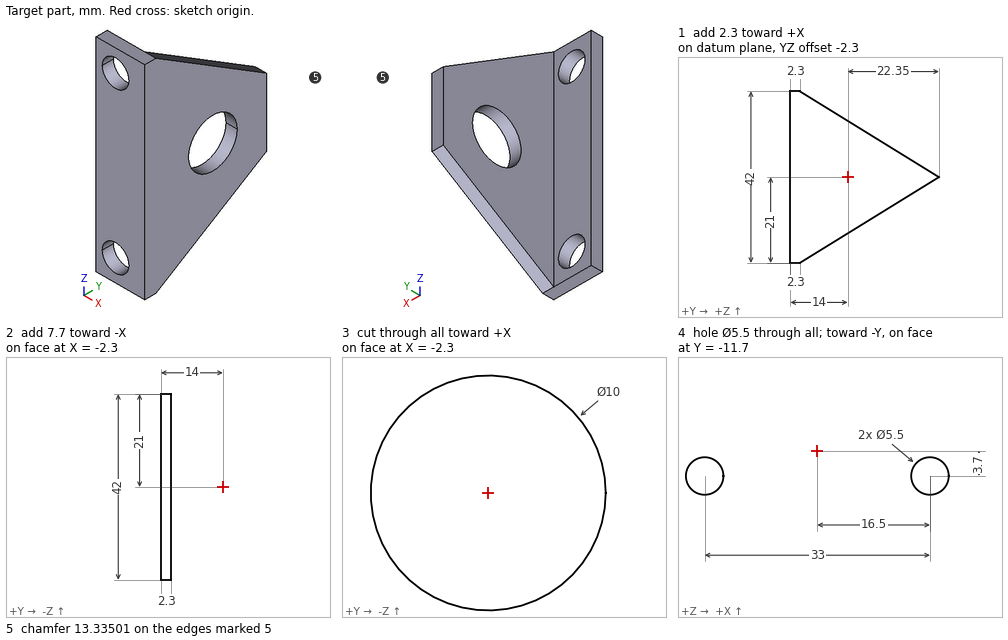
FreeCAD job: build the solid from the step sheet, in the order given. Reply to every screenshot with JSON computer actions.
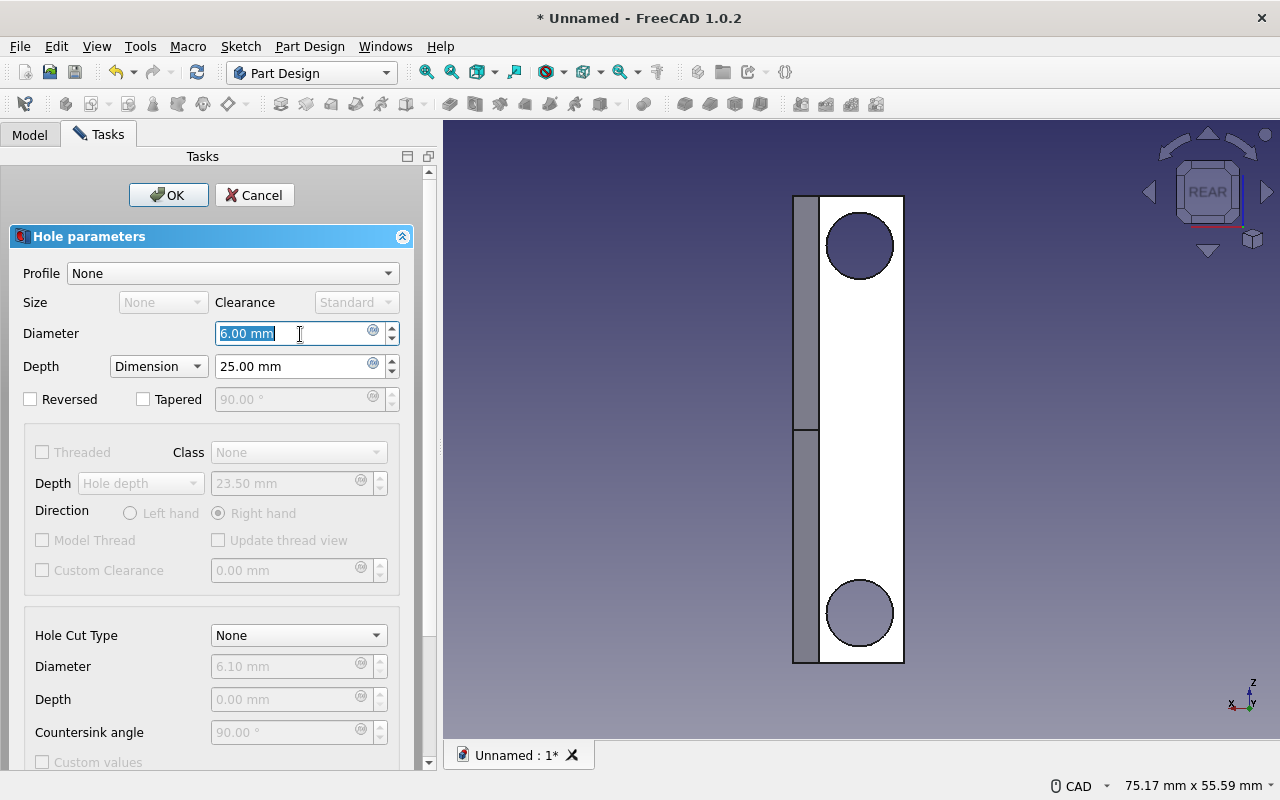
{"action": "type", "text": "5.5"}
{"action": "key", "text": "Tab"}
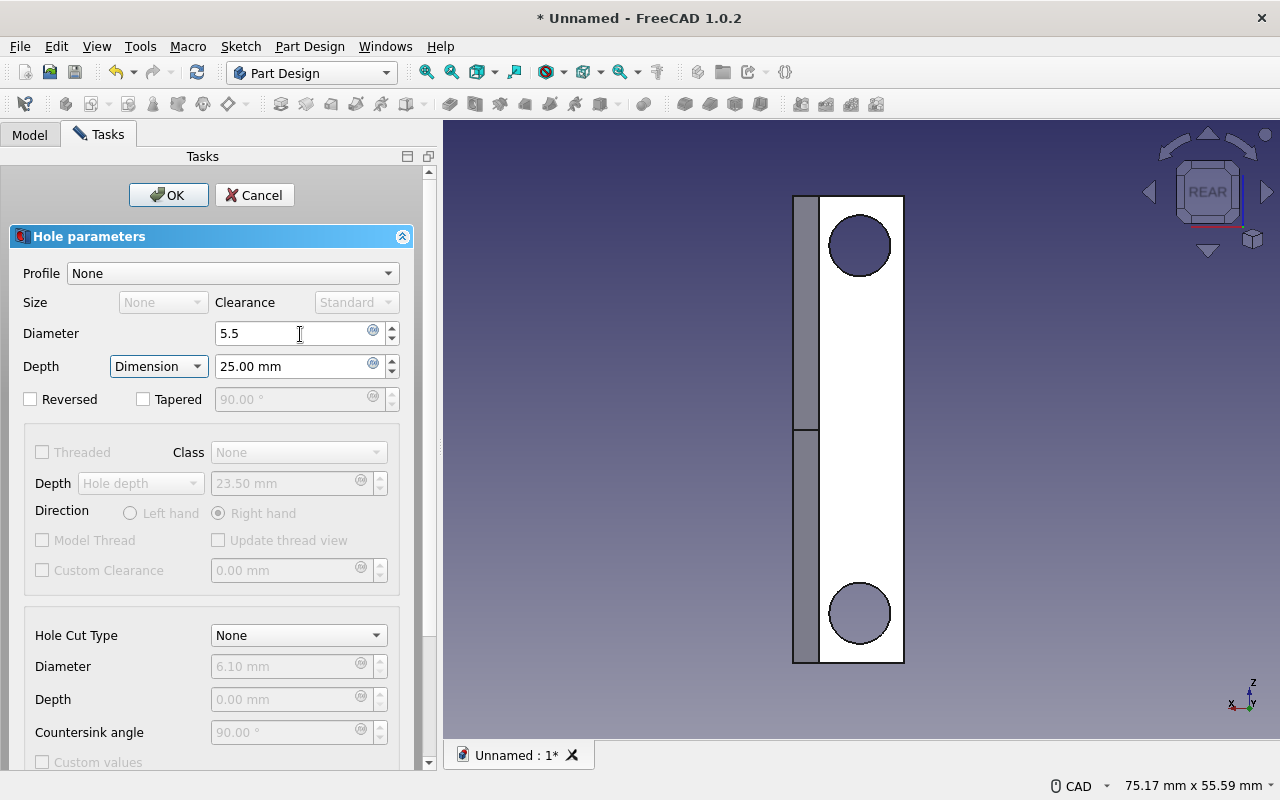
{"action": "left_click", "coordinate": [160, 366]}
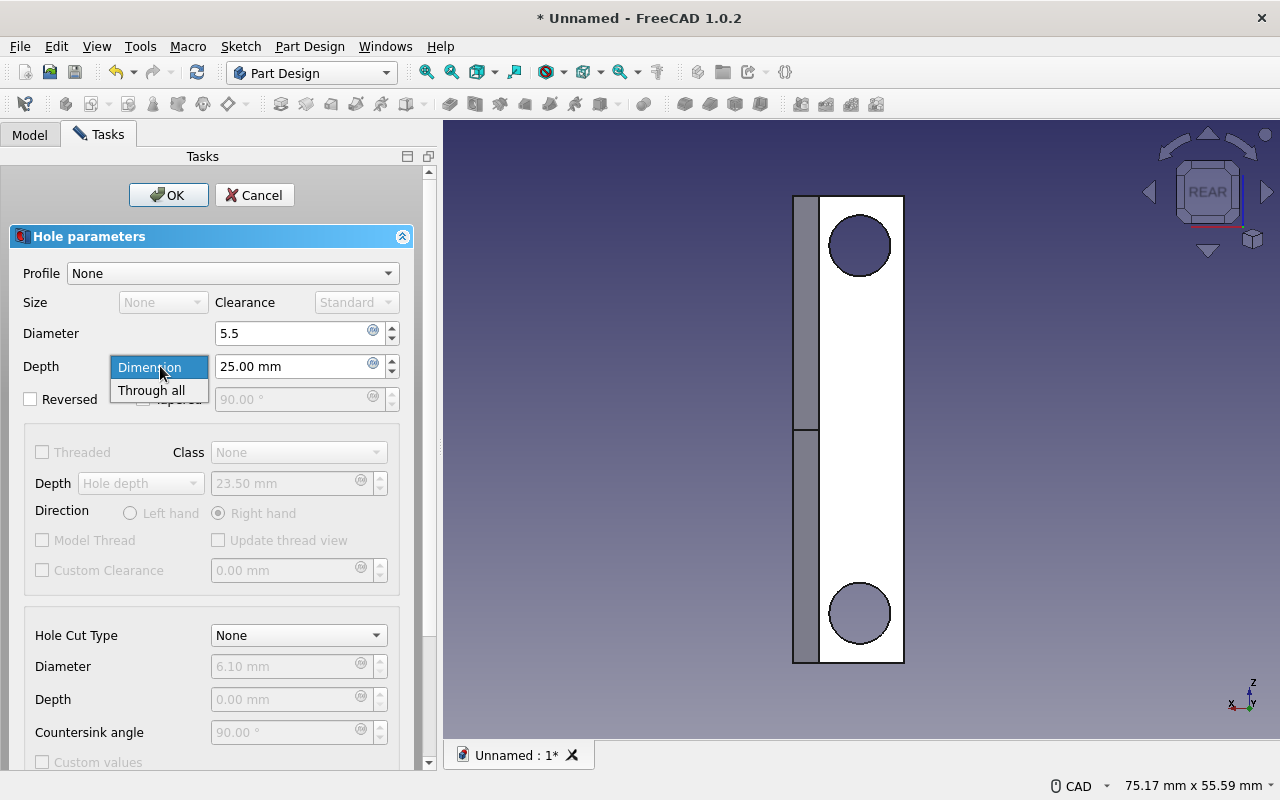
{"action": "left_click", "coordinate": [158, 390]}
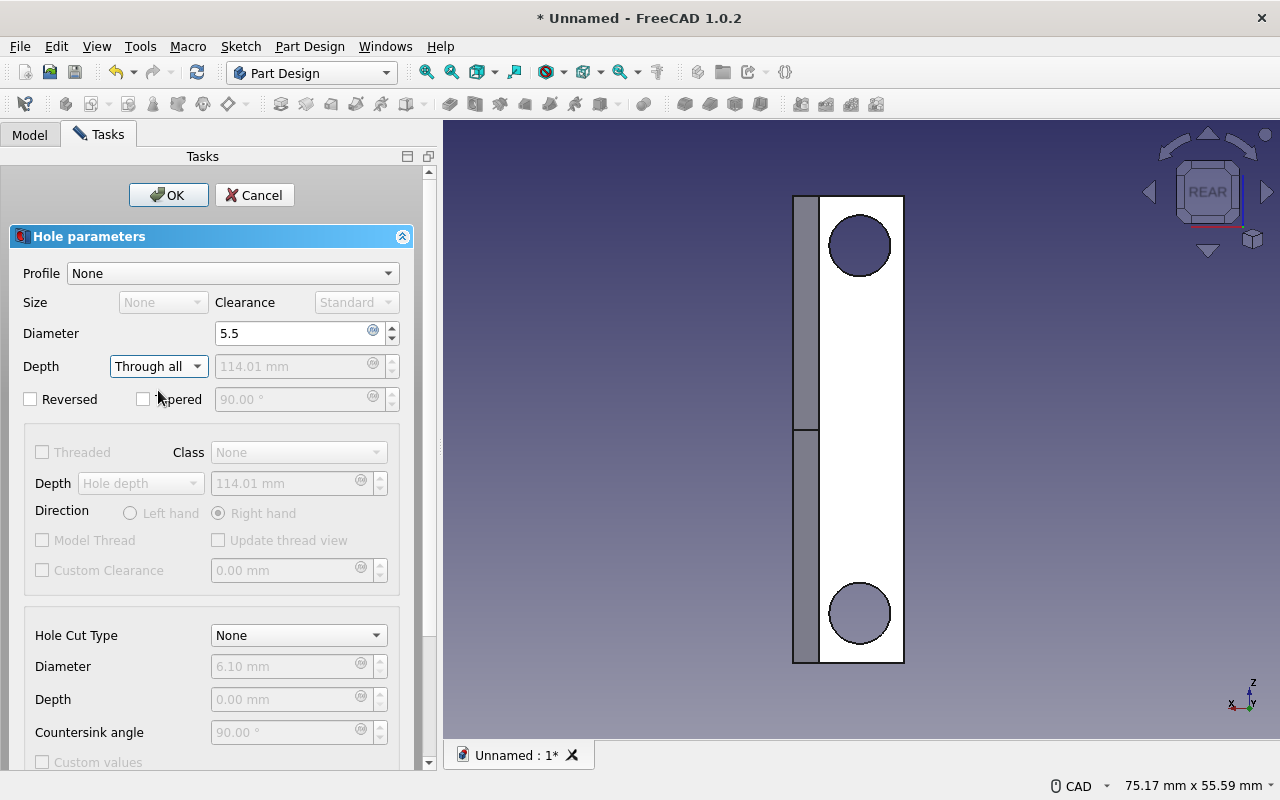
{"action": "left_click", "coordinate": [169, 195]}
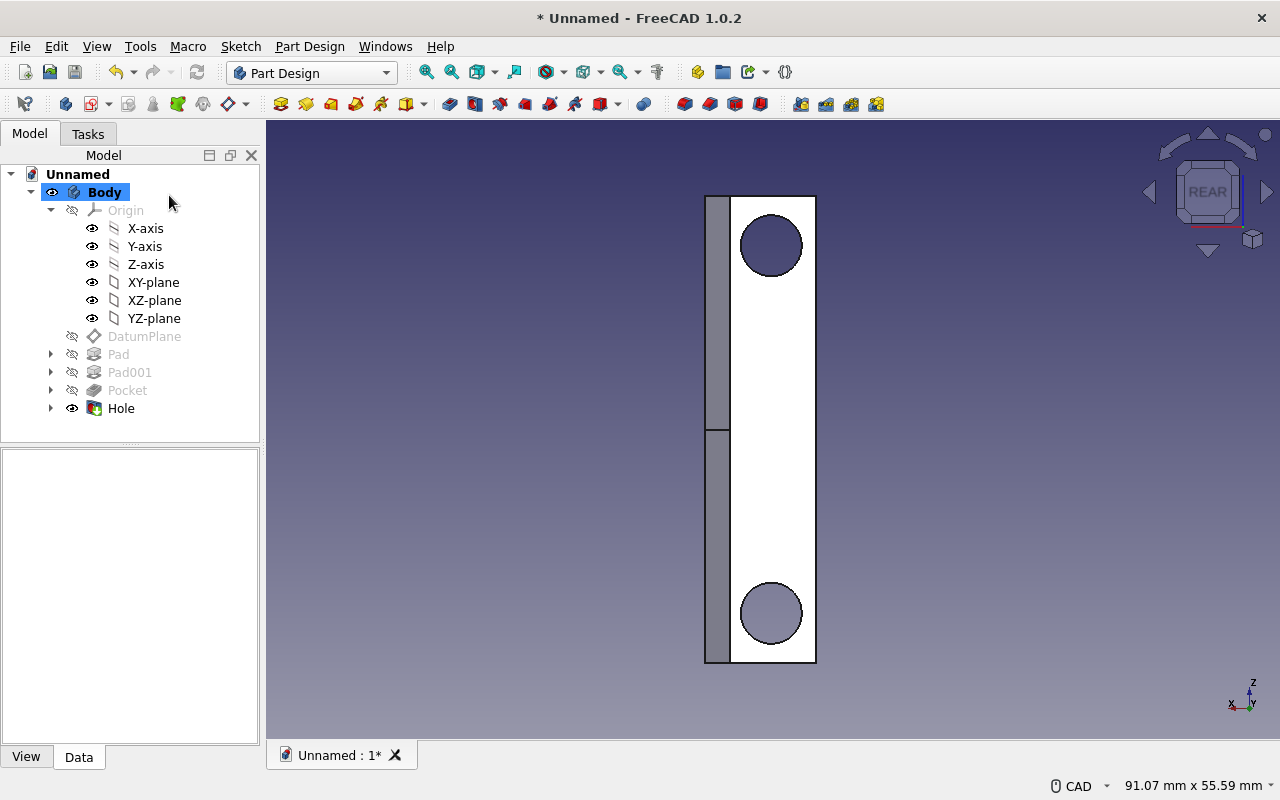
{"action": "left_click", "coordinate": [717, 429]}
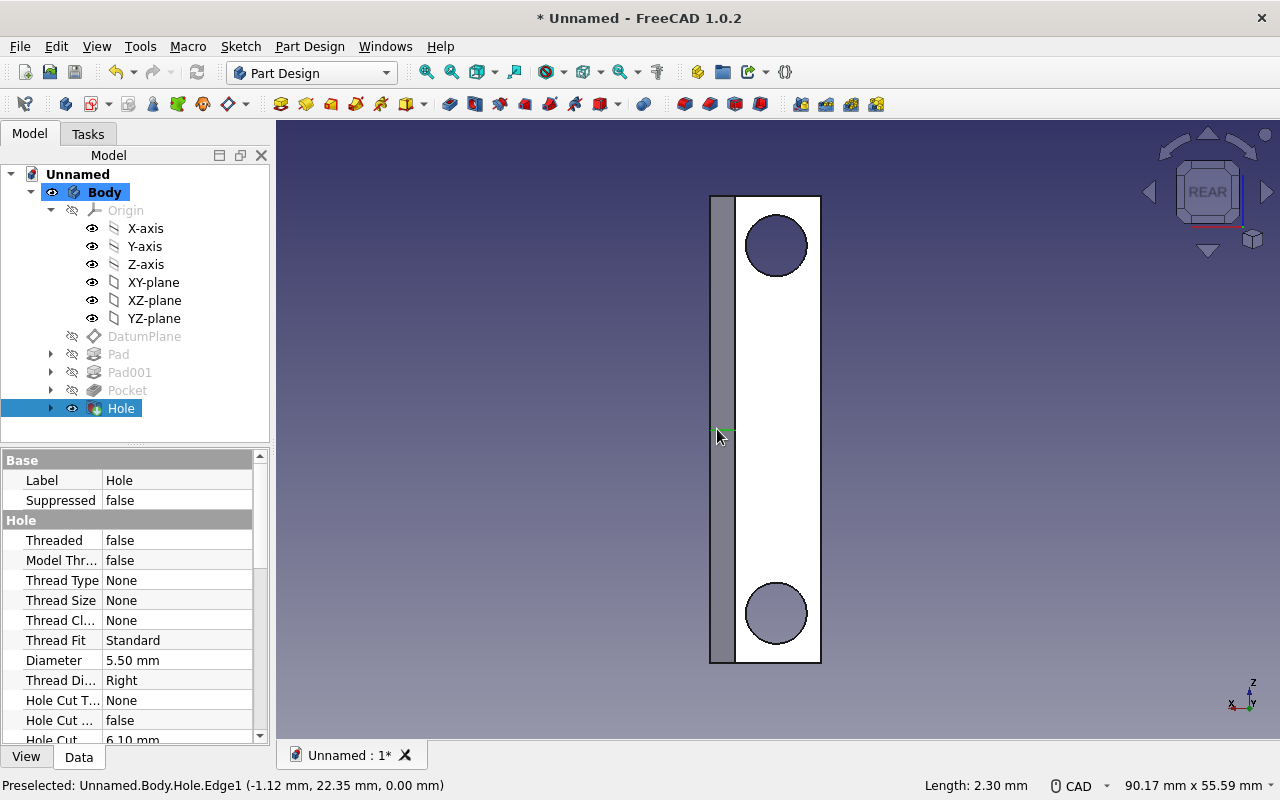
{"action": "left_click", "coordinate": [710, 104]}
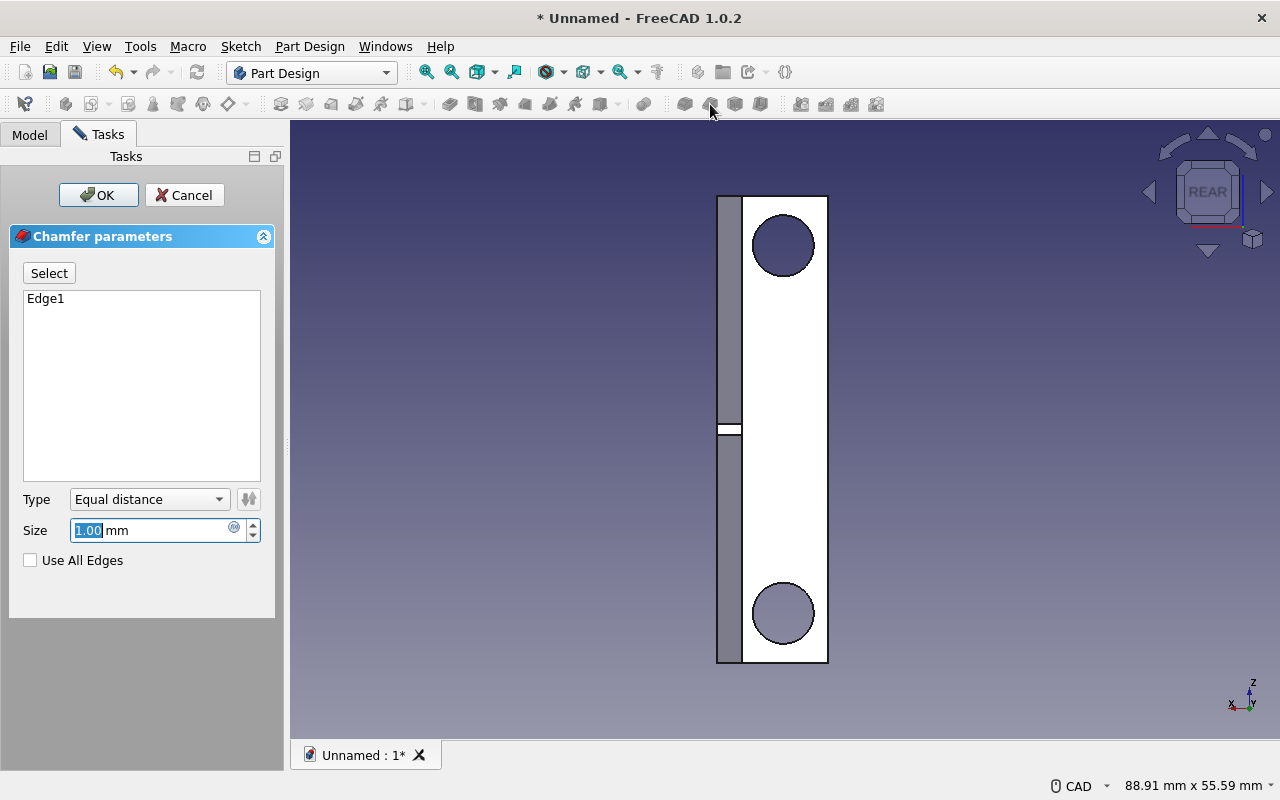
{"action": "type", "text": "13.33501"}
{"action": "key", "text": "Tab"}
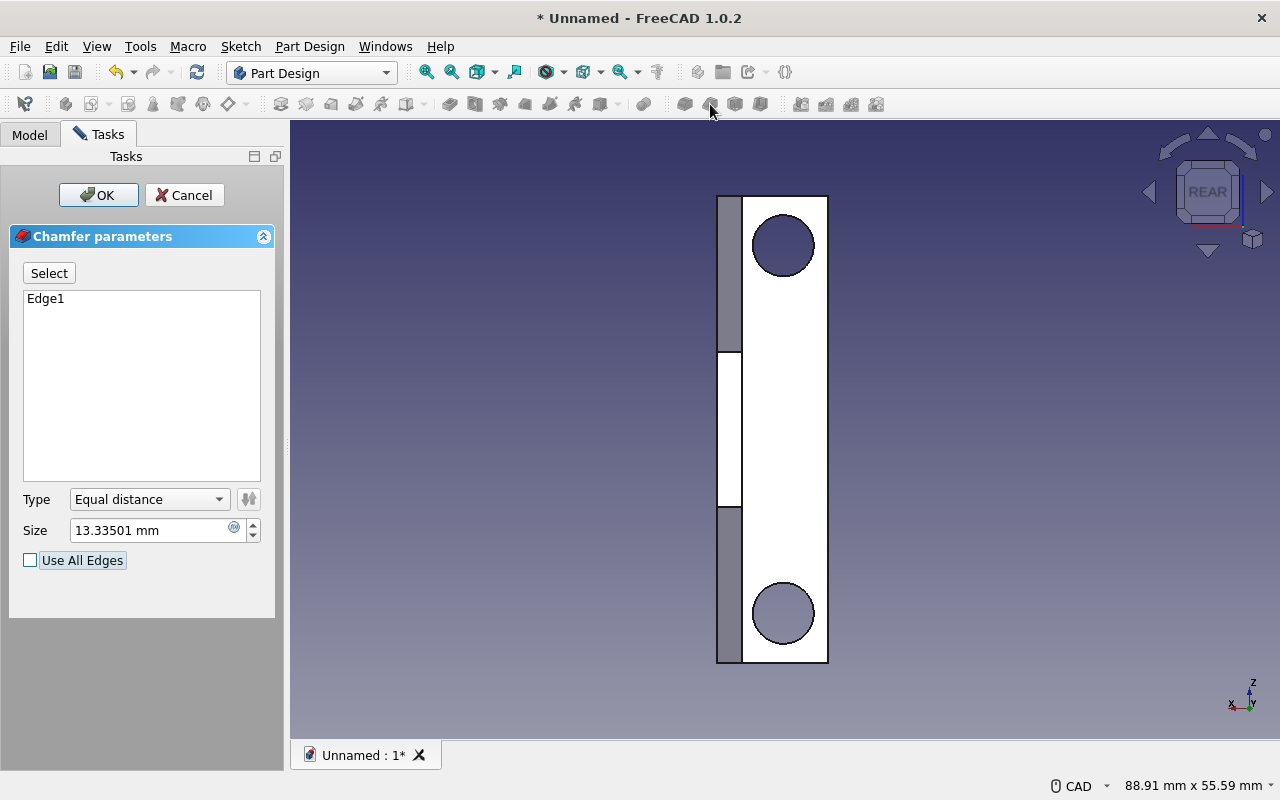
{"action": "left_click", "coordinate": [99, 195]}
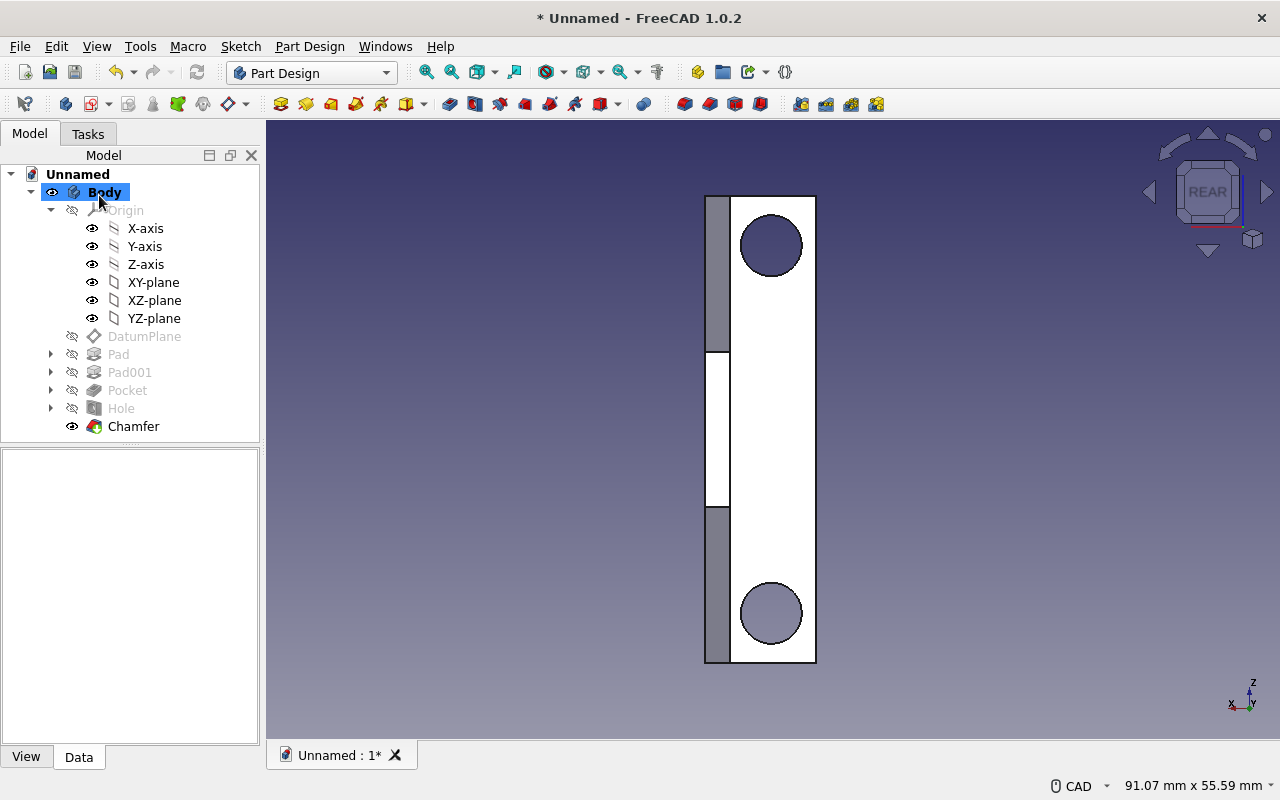
{"action": "key", "text": "0"}